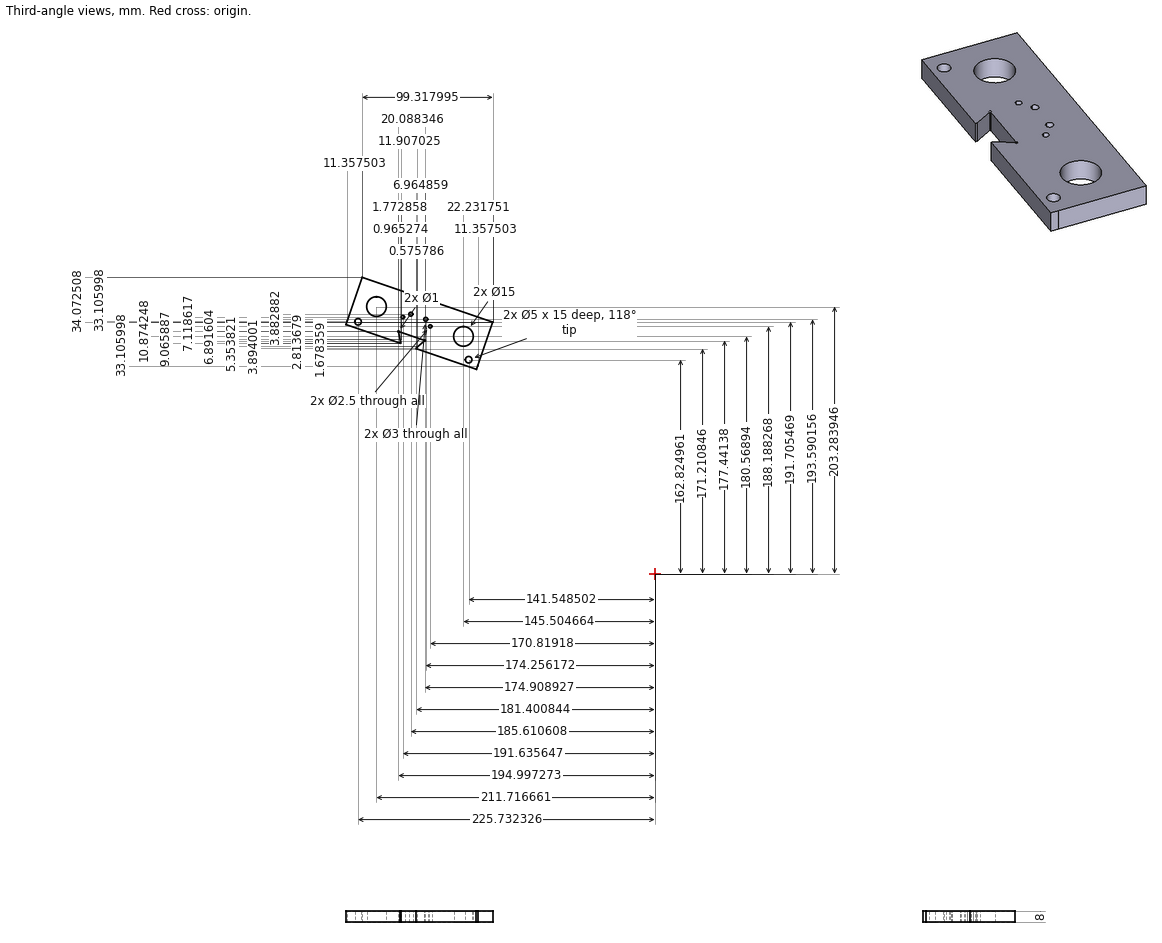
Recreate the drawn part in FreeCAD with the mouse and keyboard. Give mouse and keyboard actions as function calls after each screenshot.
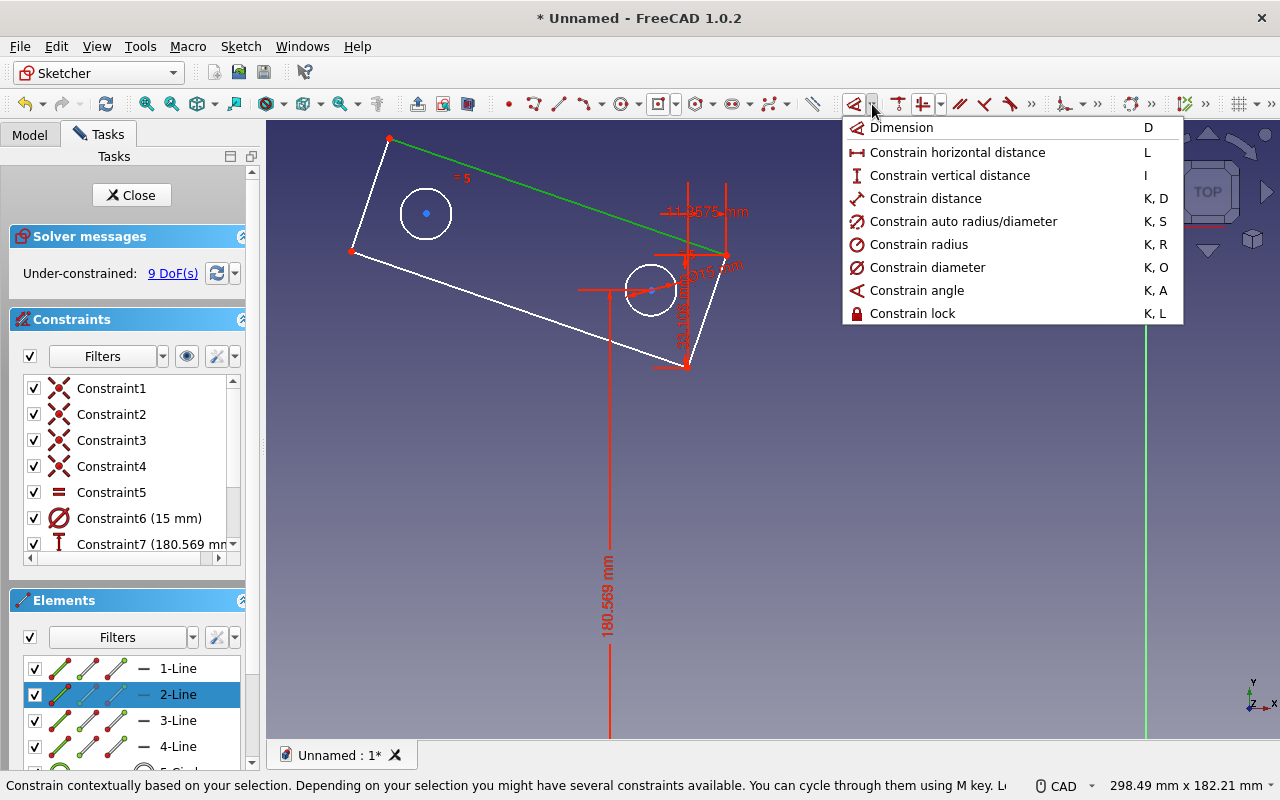
click(1013, 152)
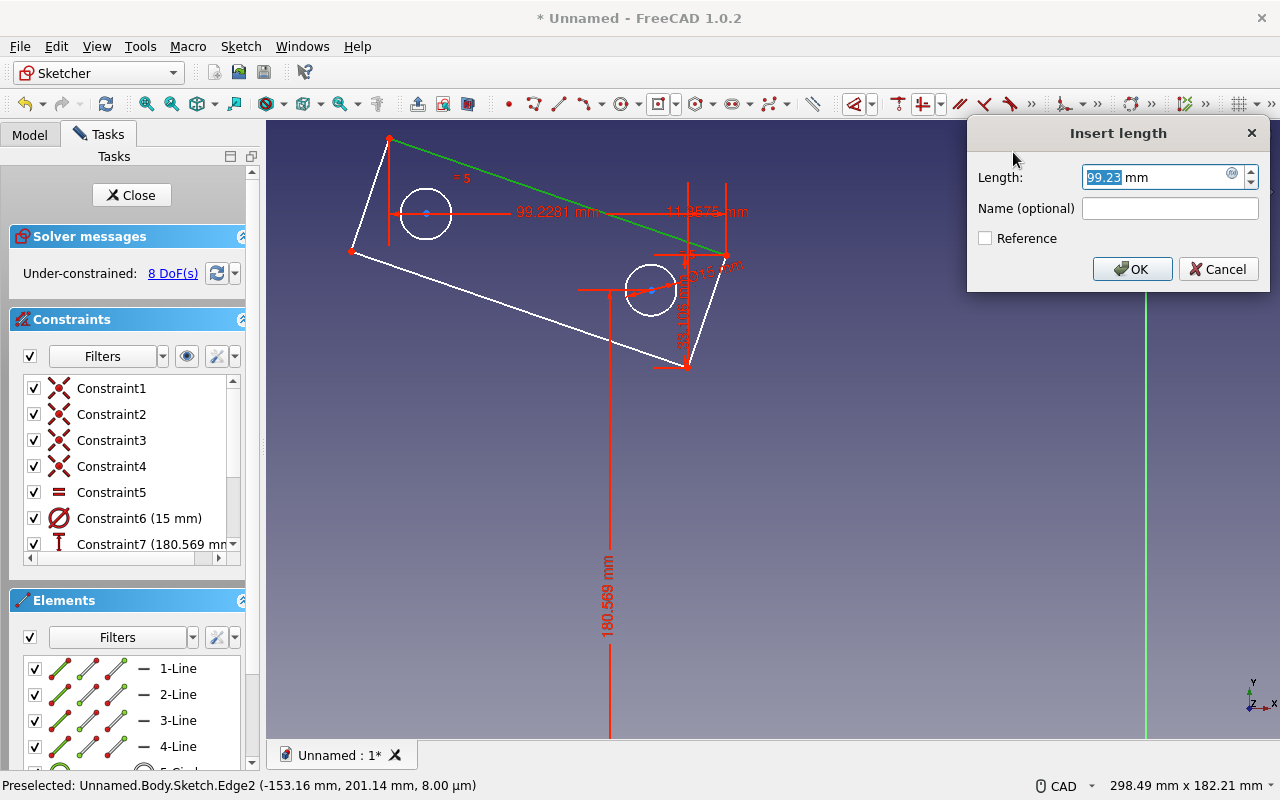
text(99.317995)
key(Return)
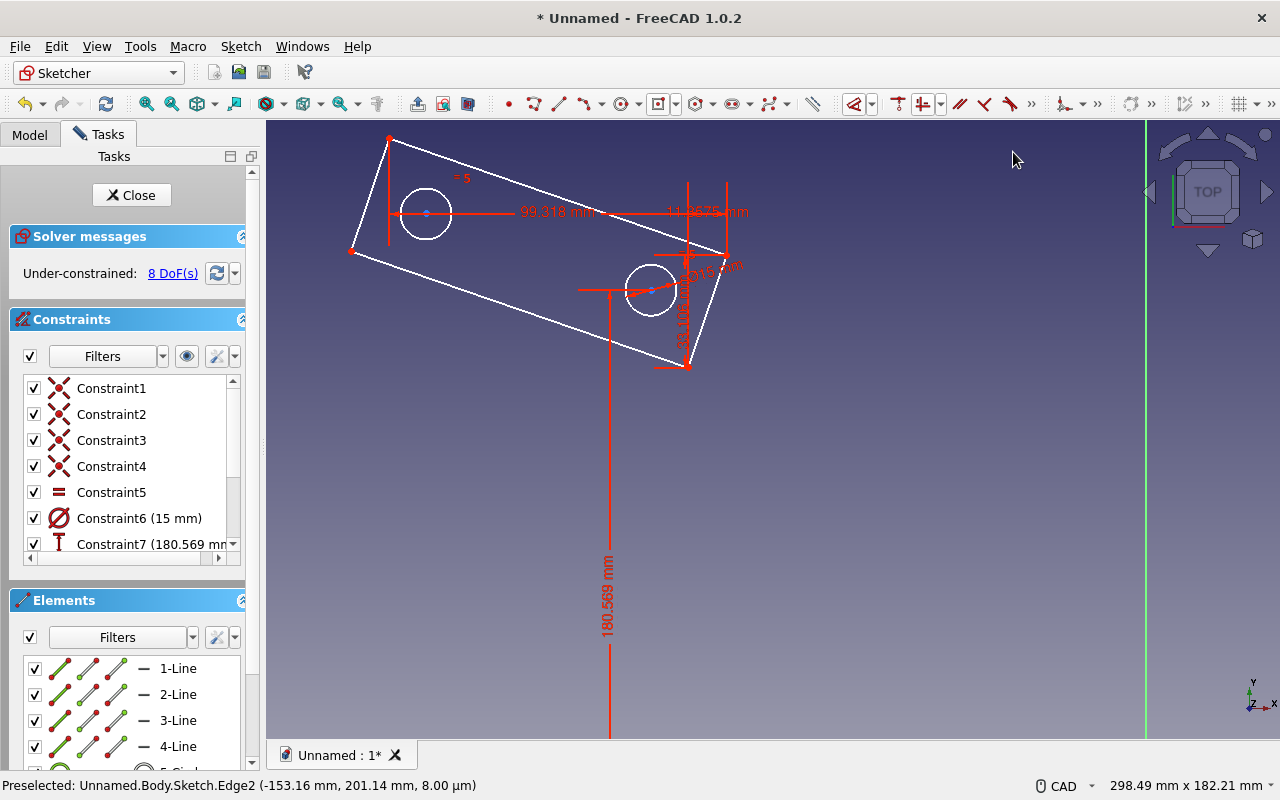
click(625, 220)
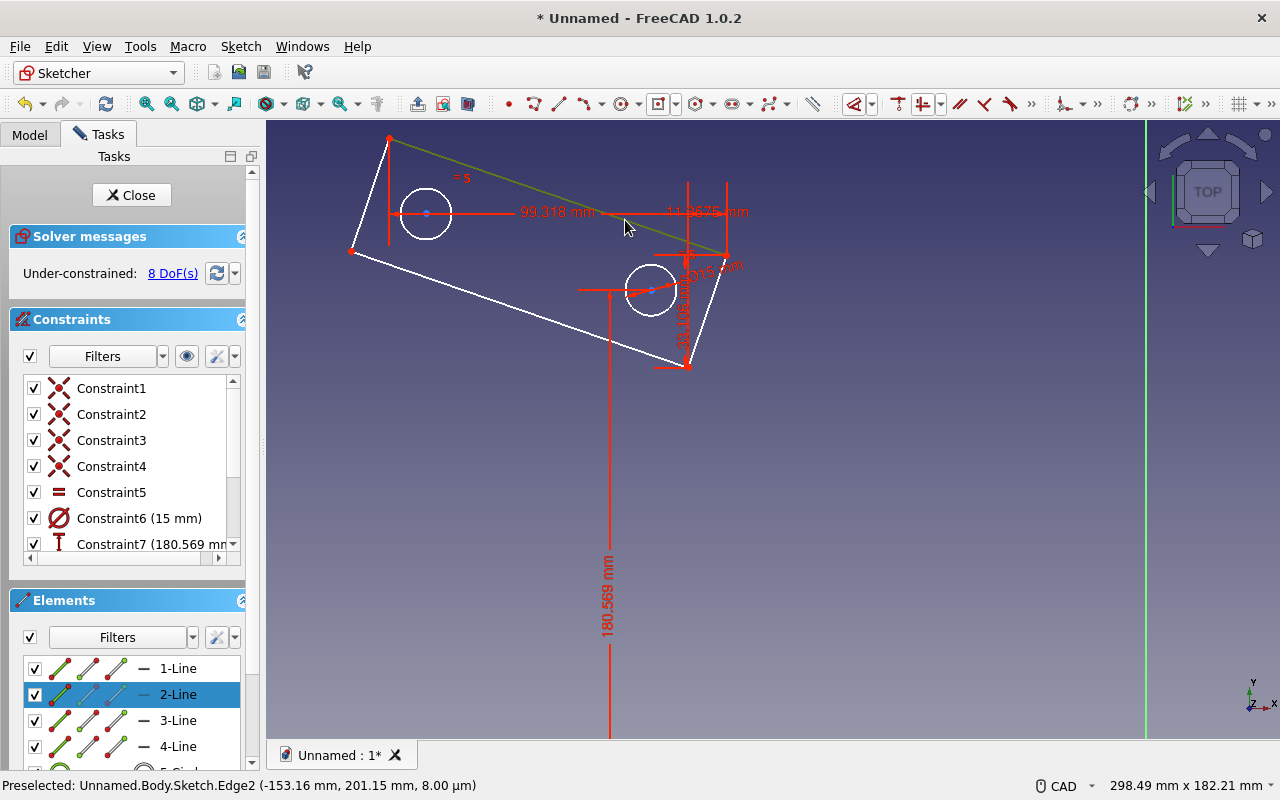
click(872, 104)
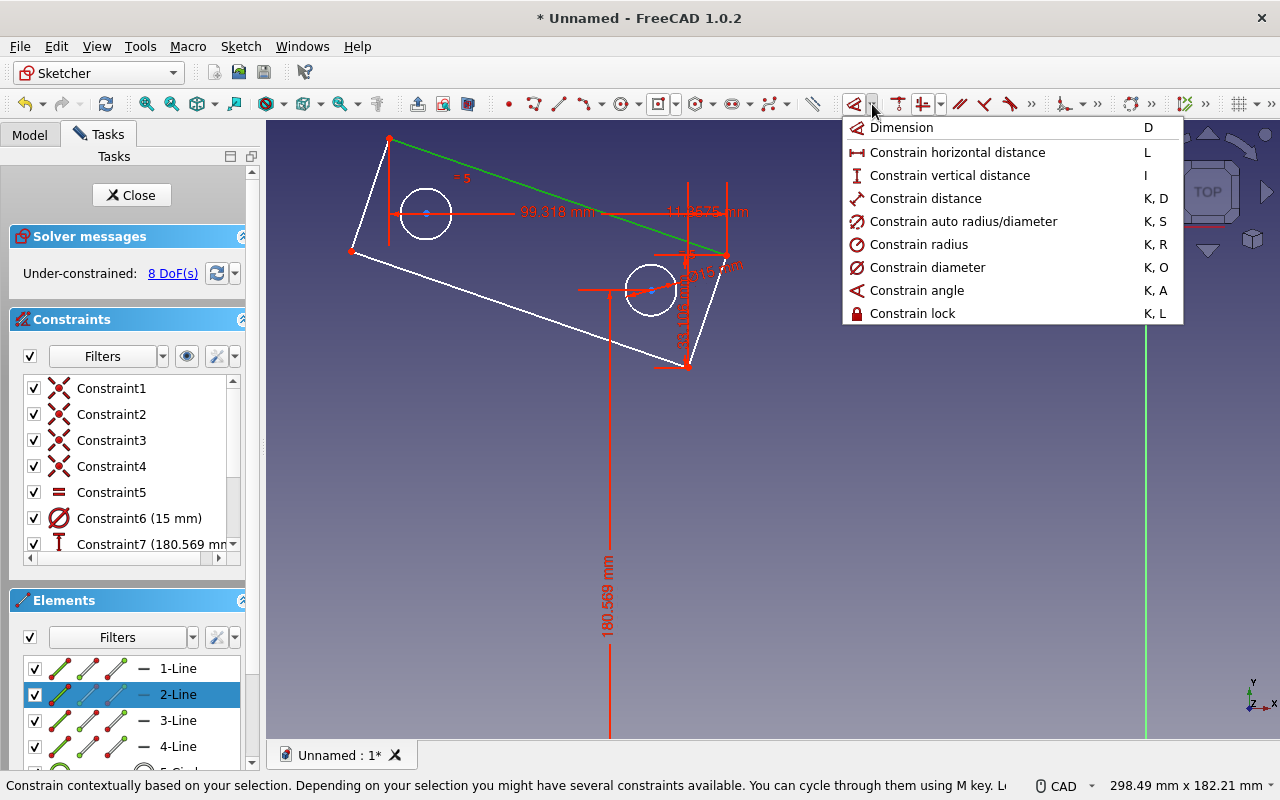
click(1013, 176)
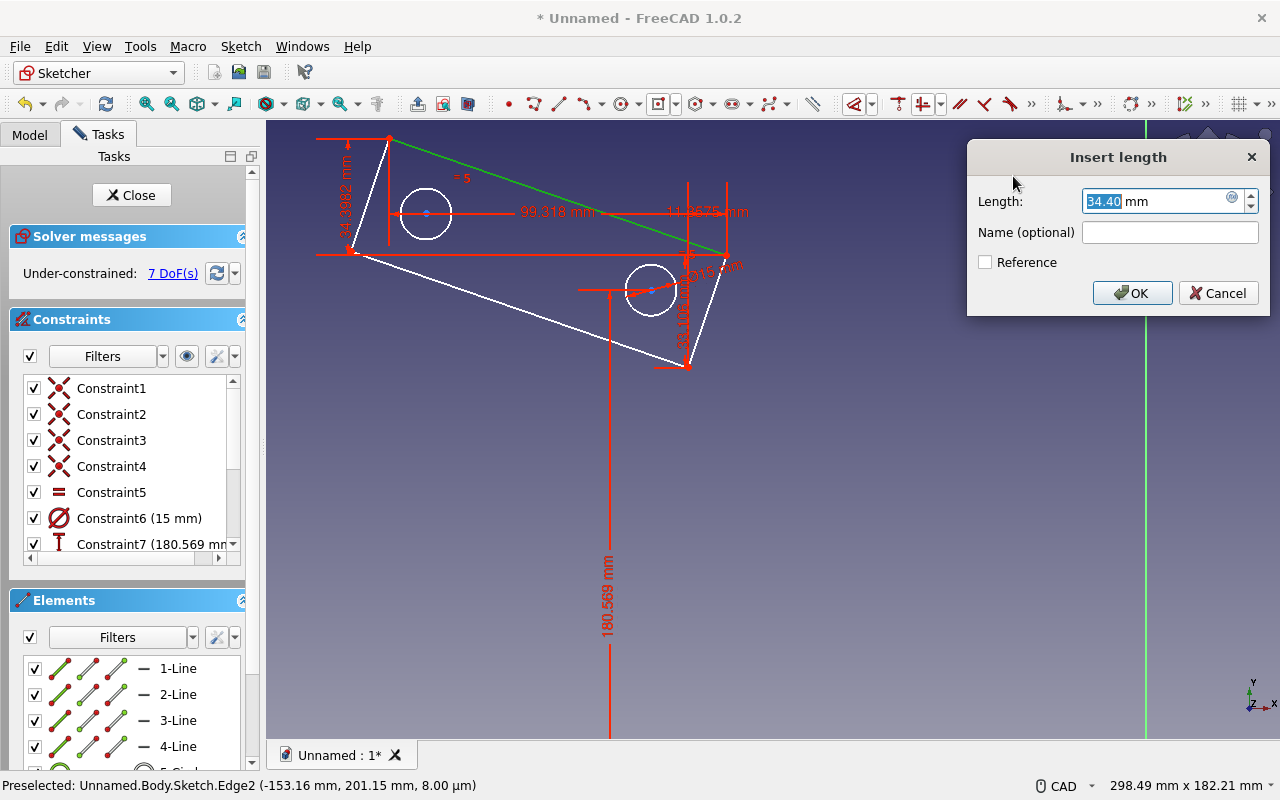
text(34.072508)
key(Return)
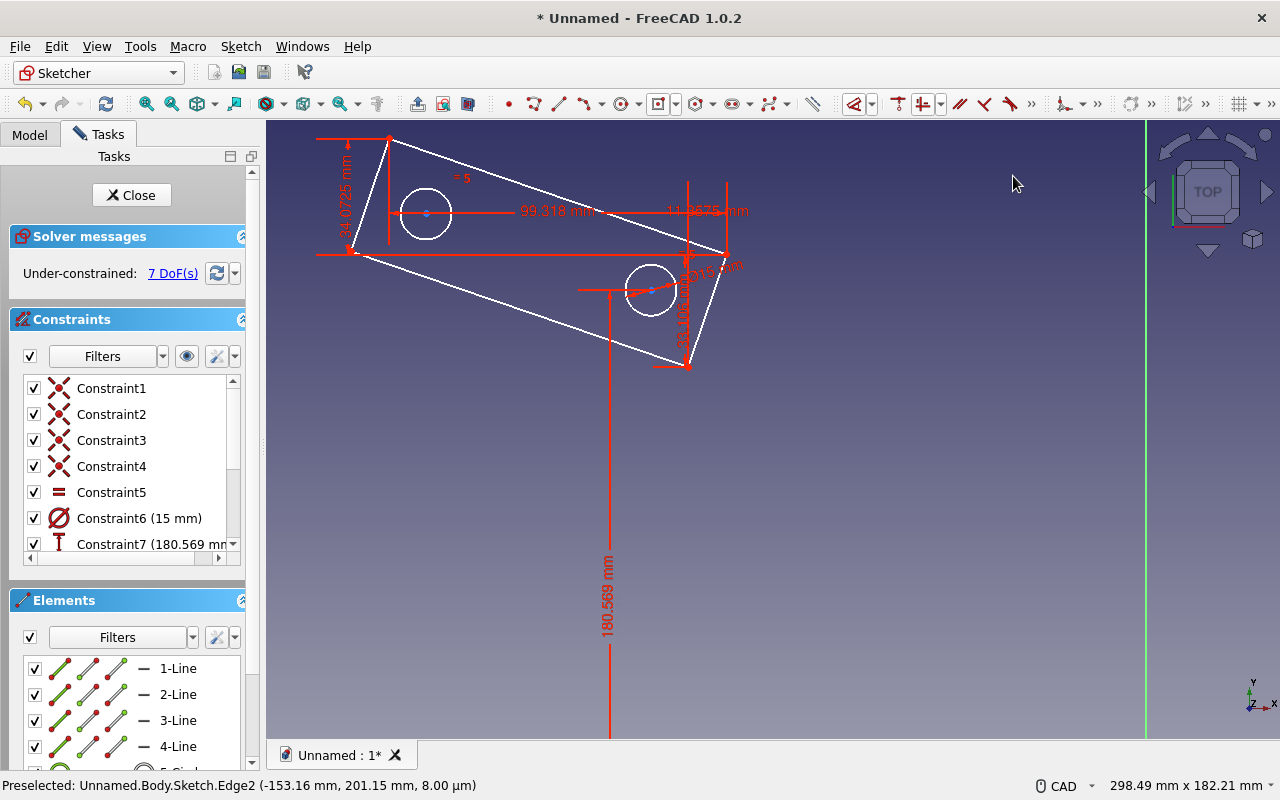
click(378, 173)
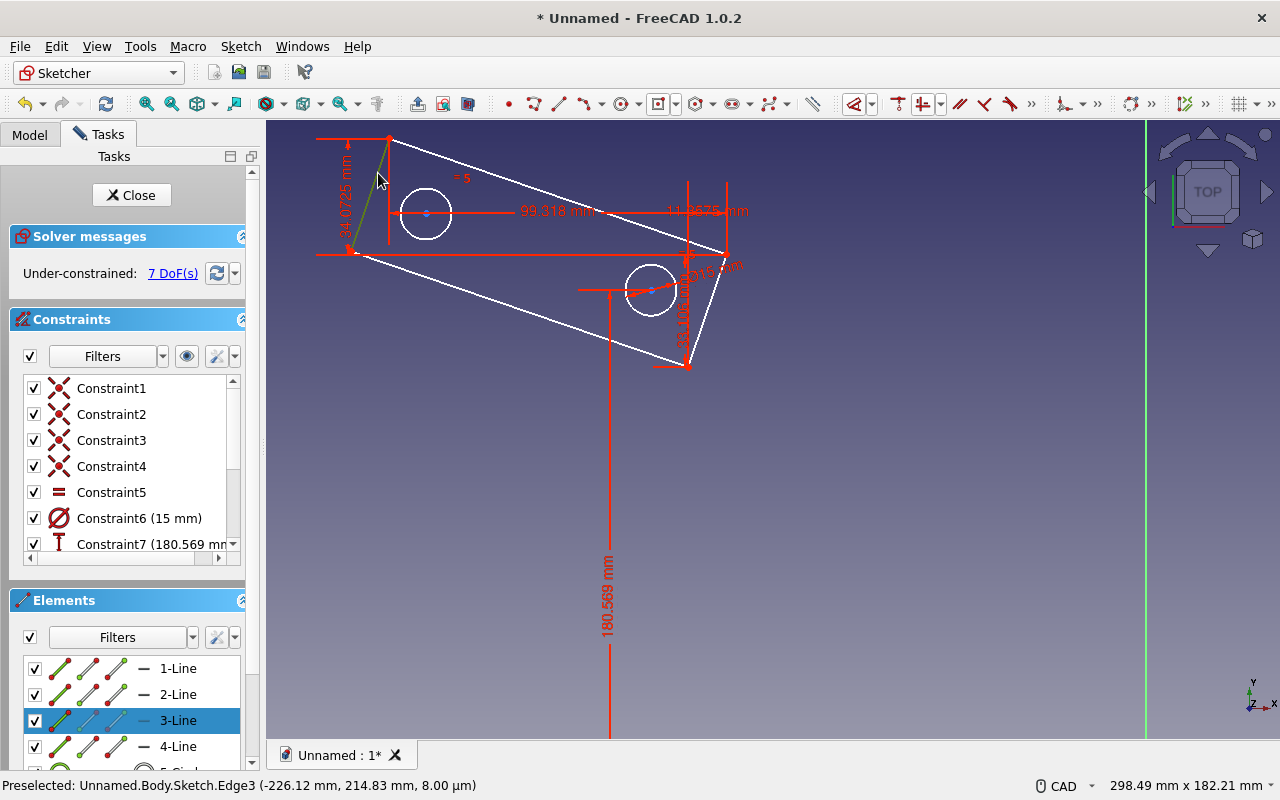
click(872, 104)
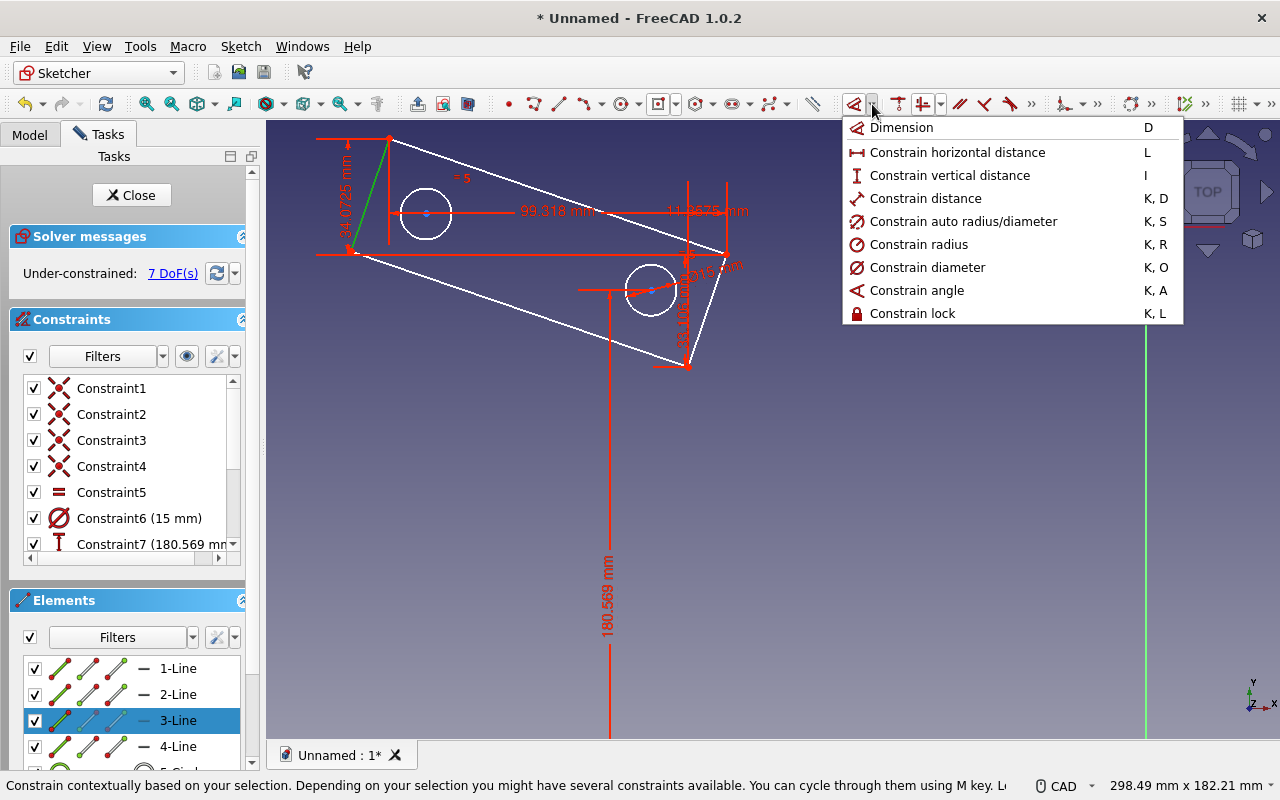
click(1013, 152)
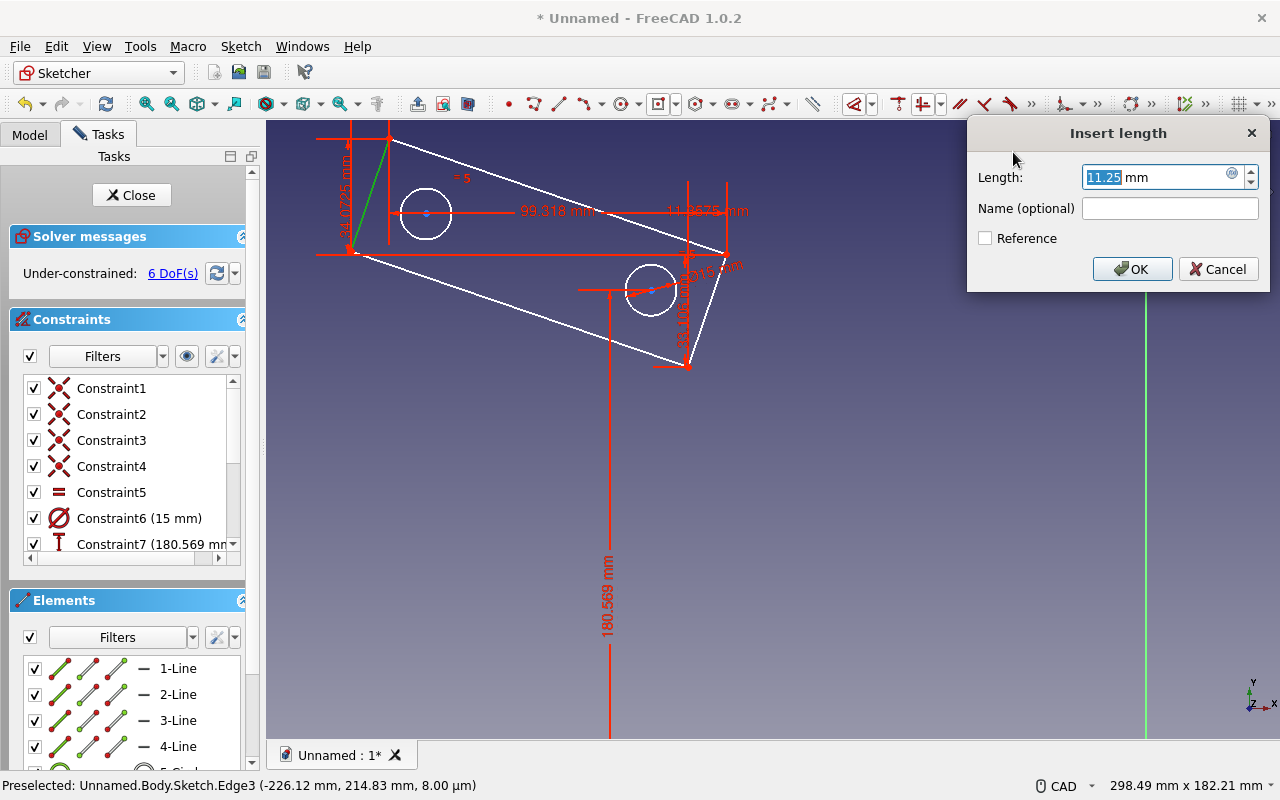
text(11.357503)
key(Return)